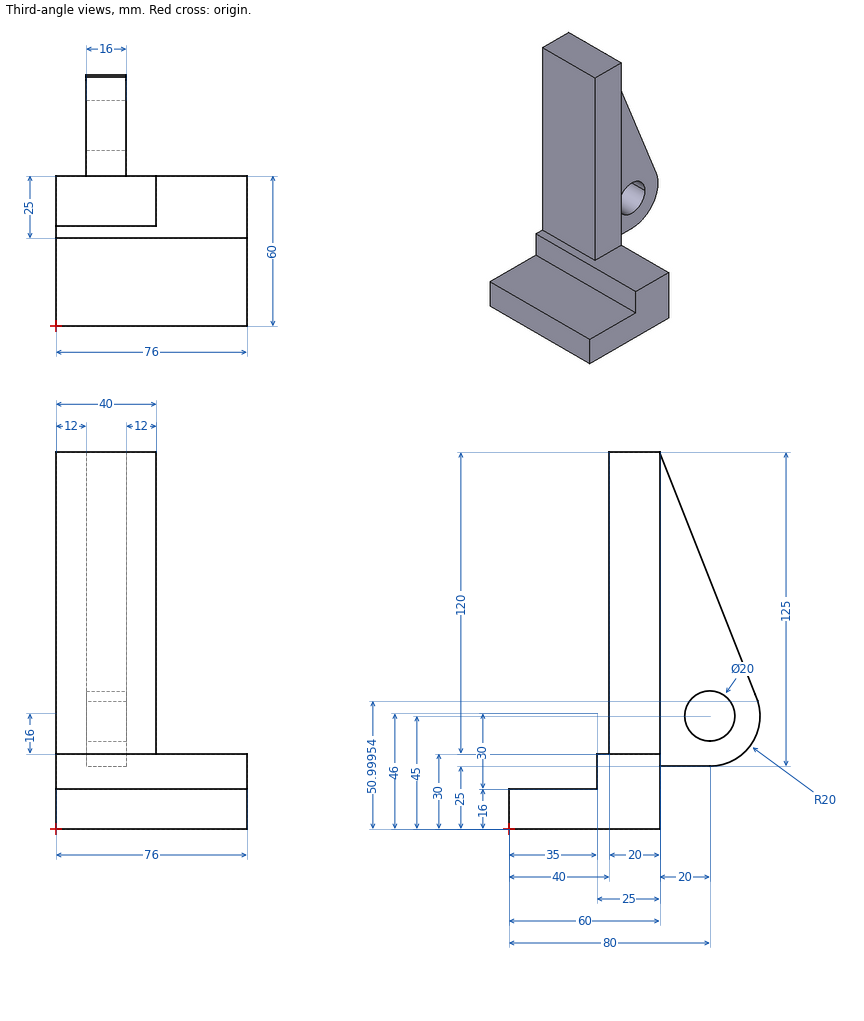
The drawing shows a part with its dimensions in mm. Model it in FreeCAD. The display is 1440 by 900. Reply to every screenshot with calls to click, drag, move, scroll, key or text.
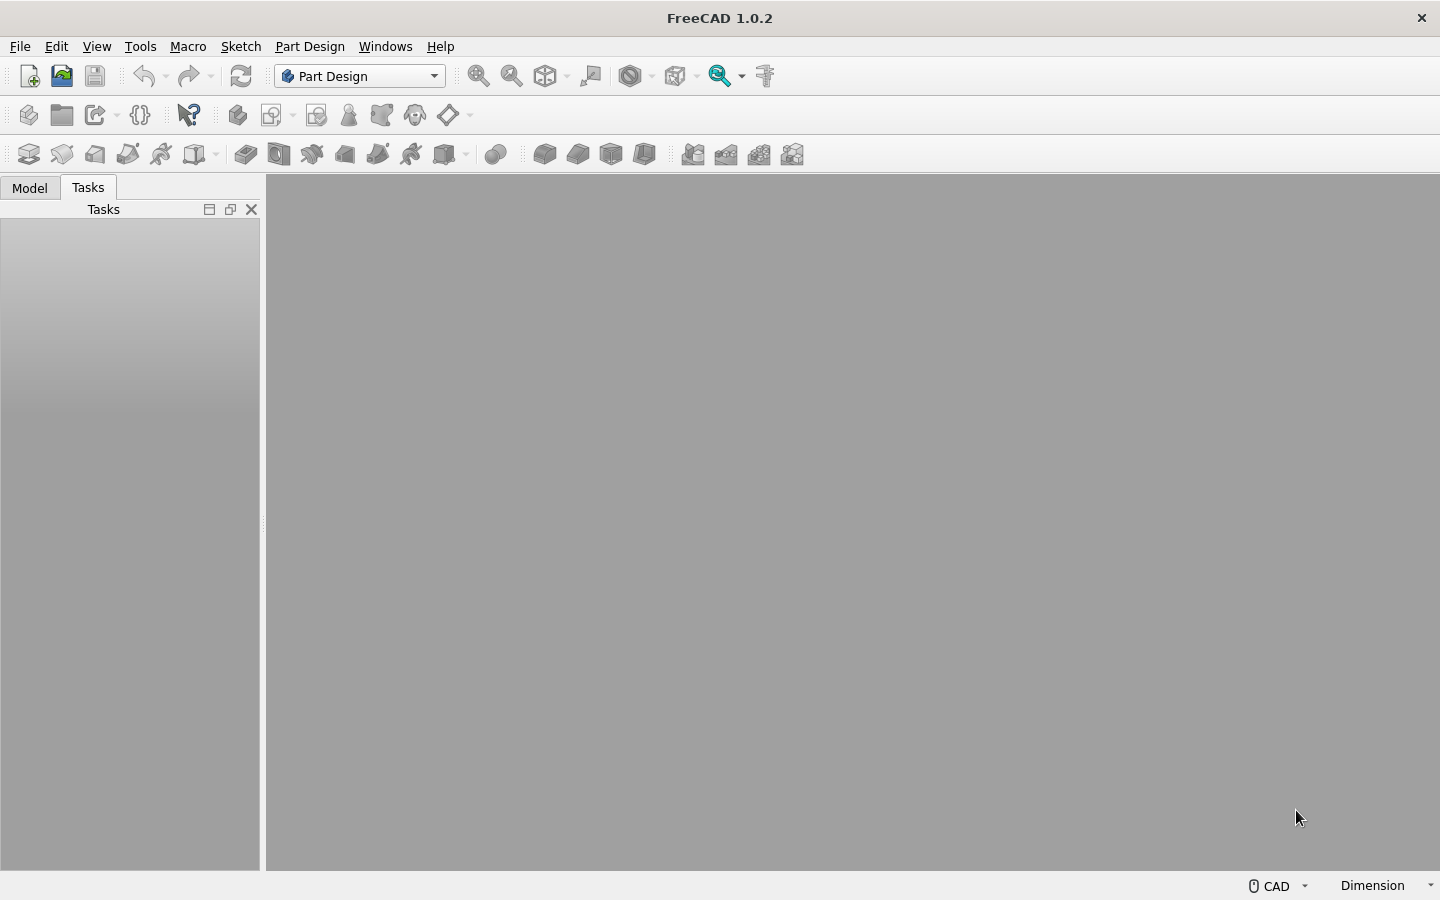
key(ctrl+n)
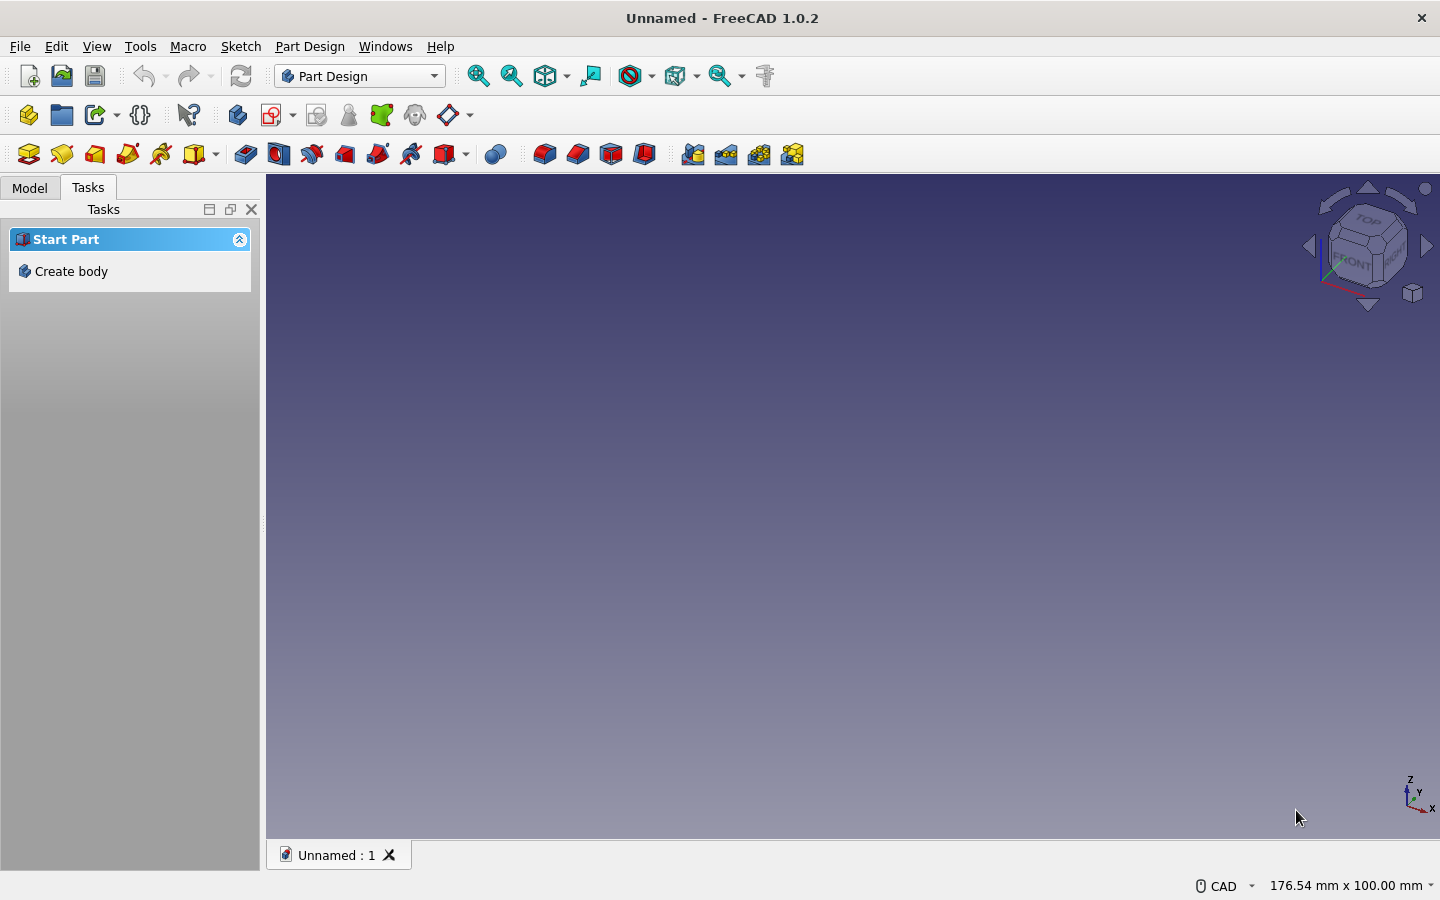
click(270, 116)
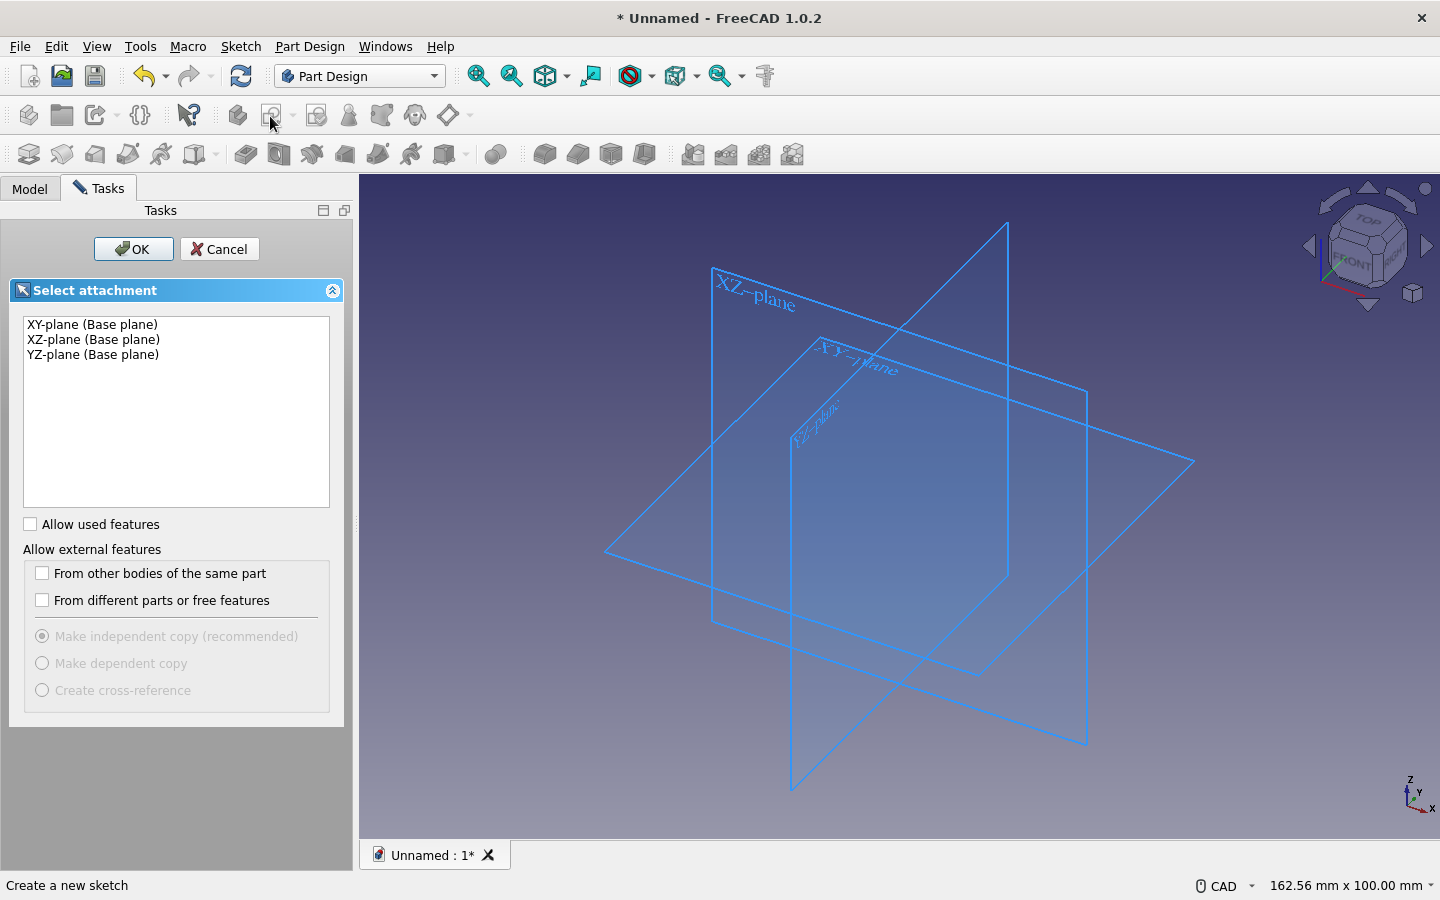
click(84, 324)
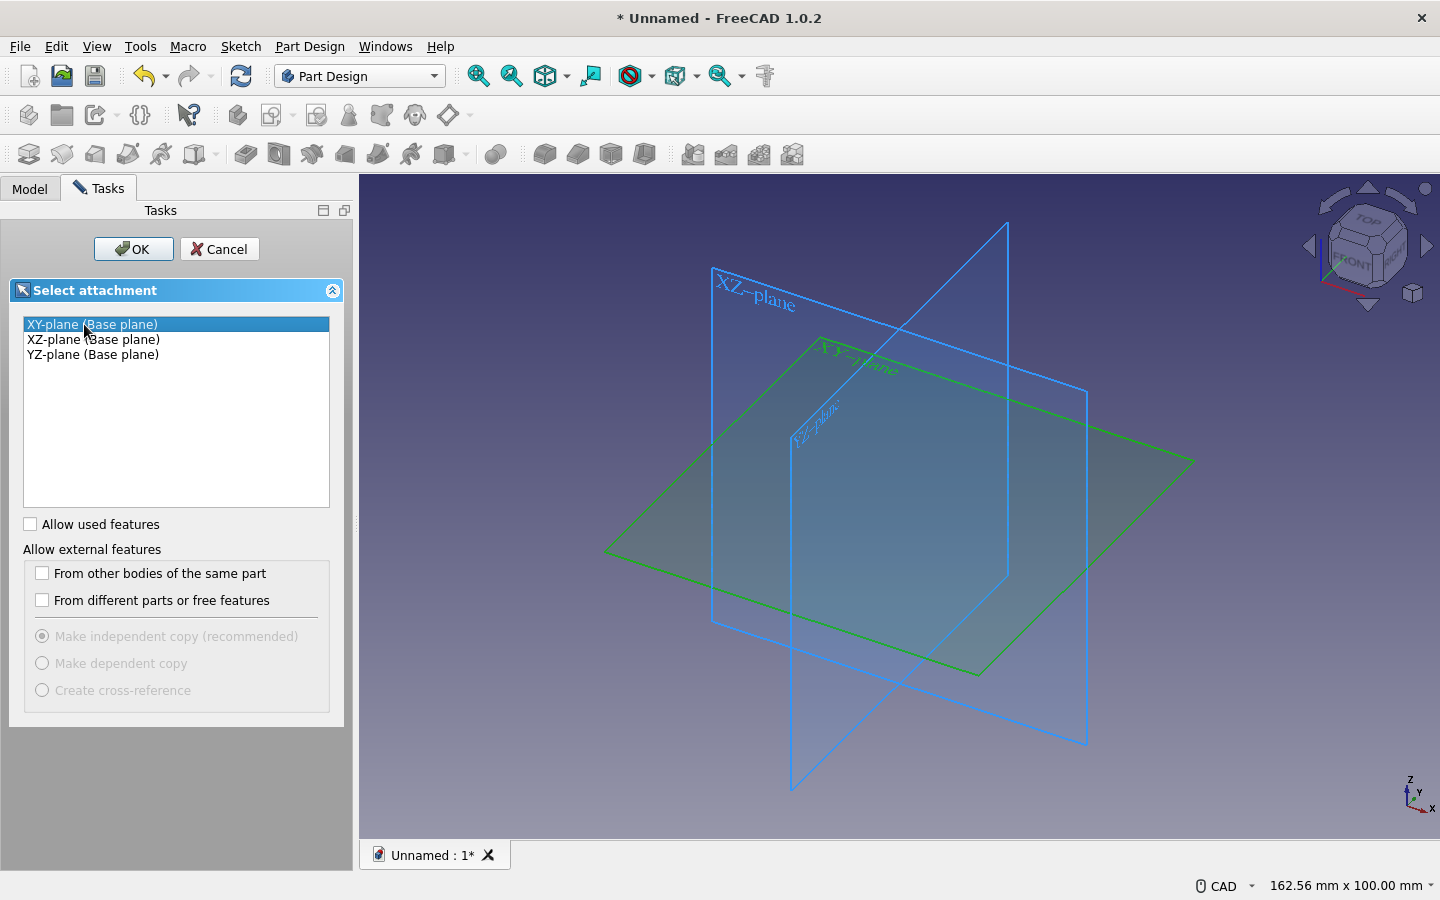
click(134, 249)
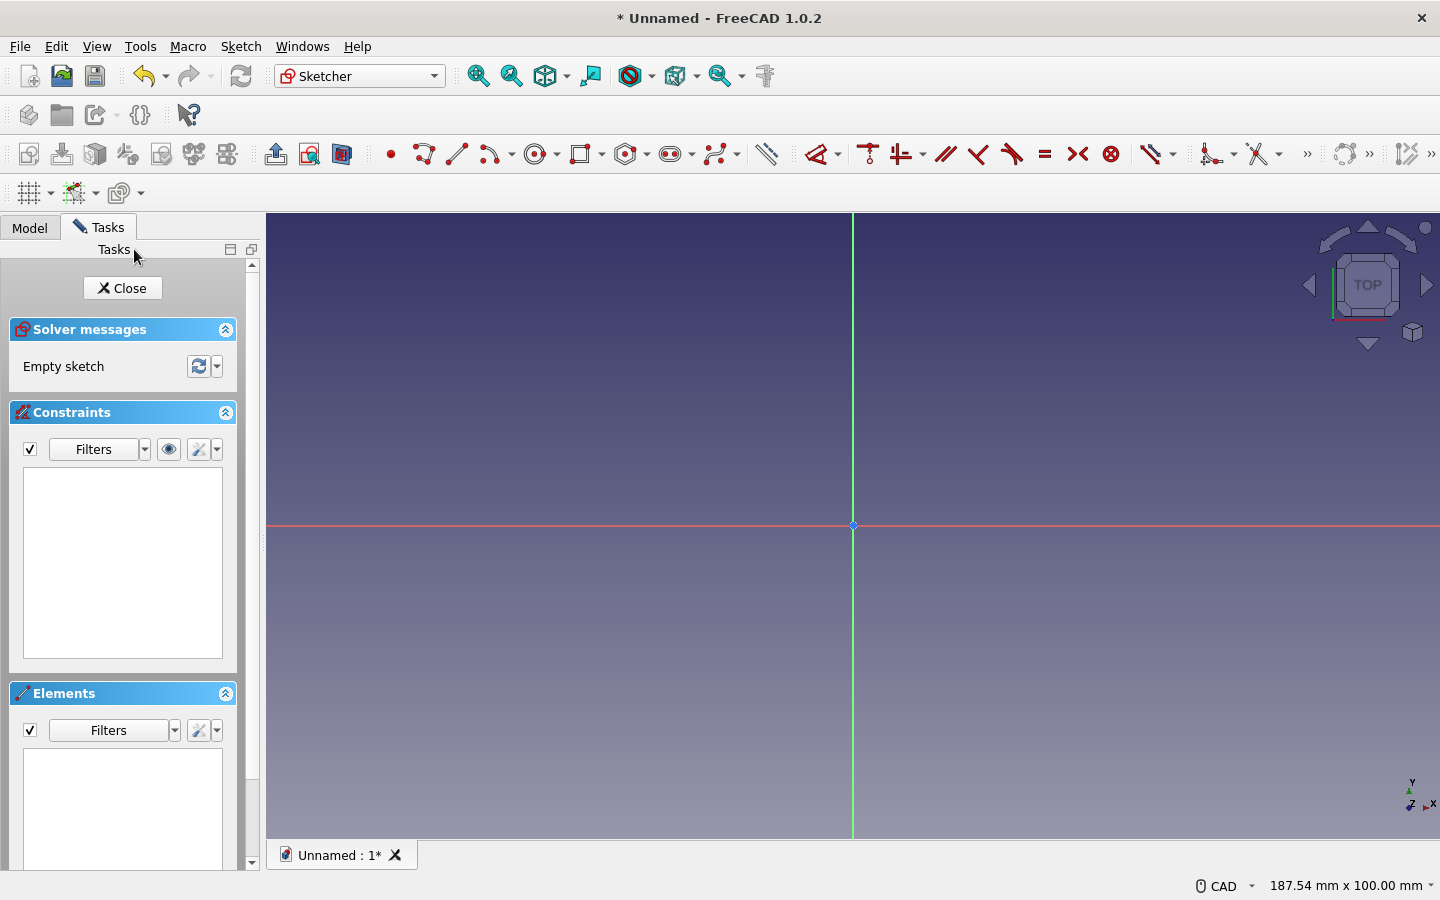
scroll(294, 811, down, 1)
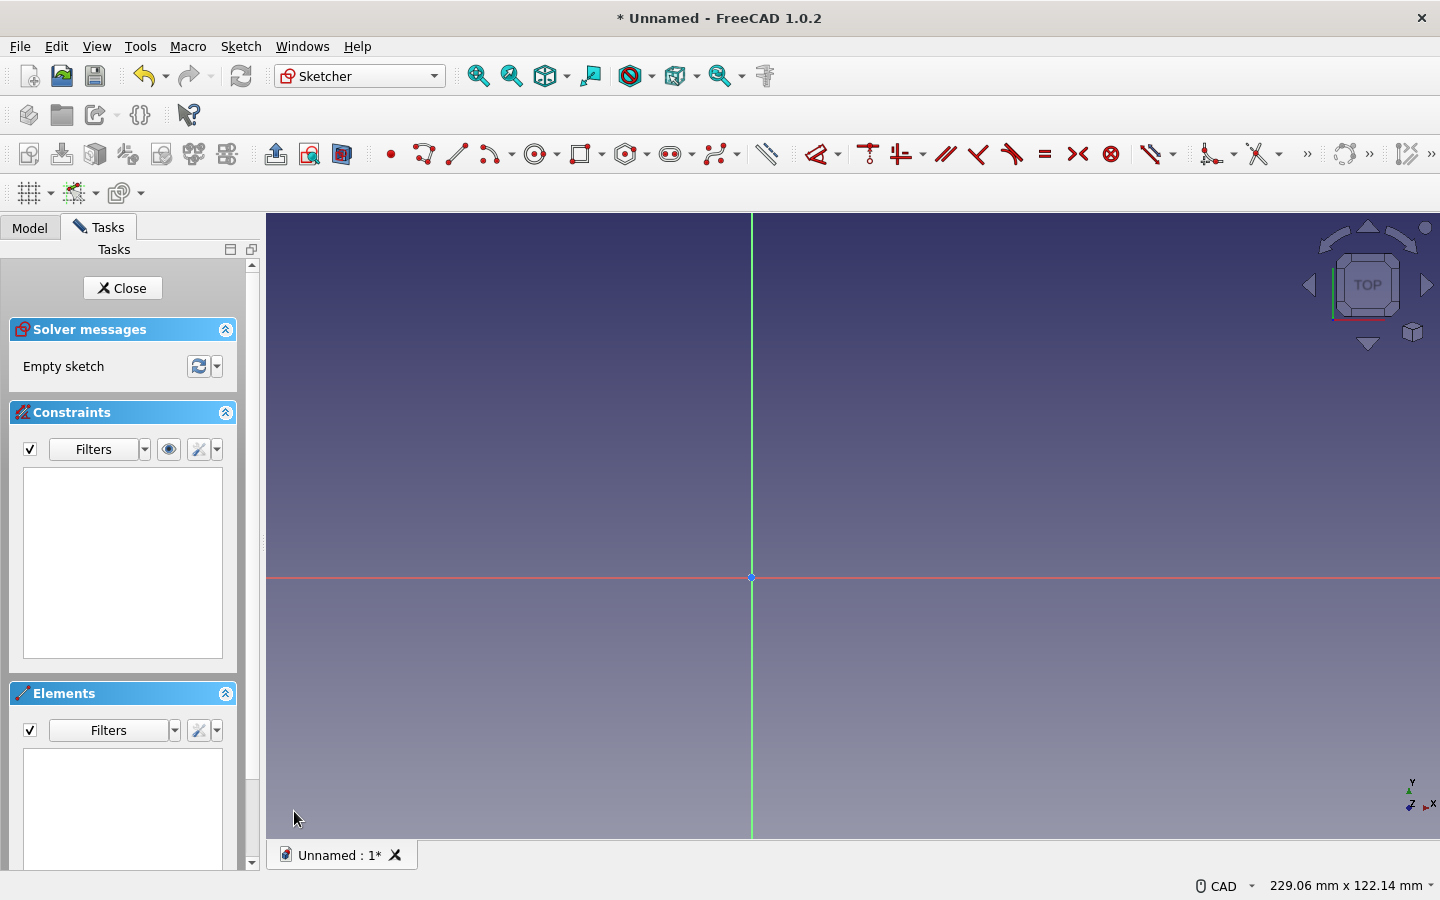
key(g)
key(r)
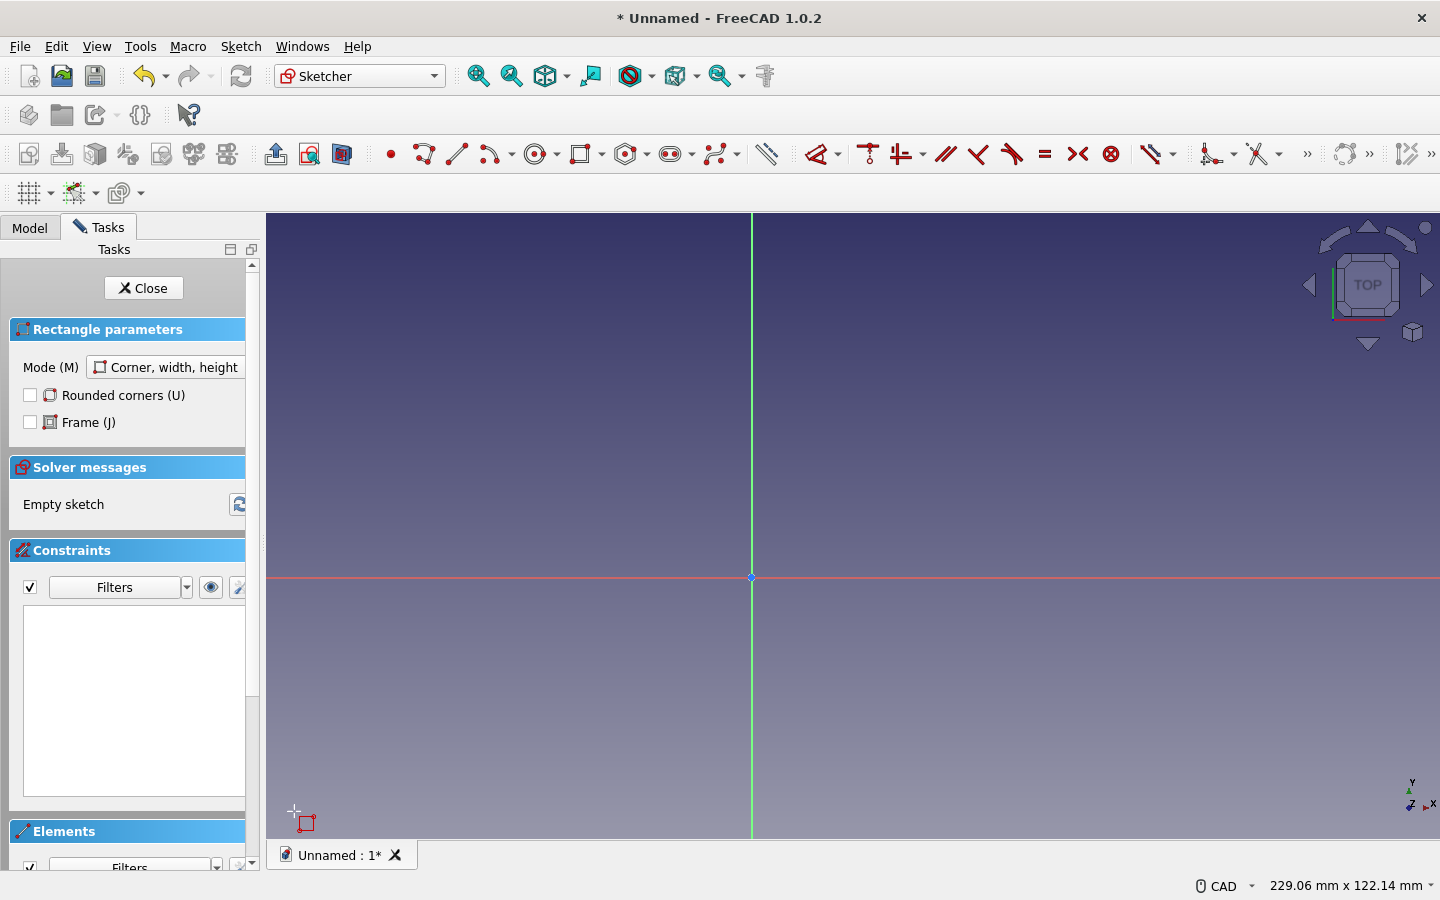
click(752, 578)
click(1141, 270)
key(Escape)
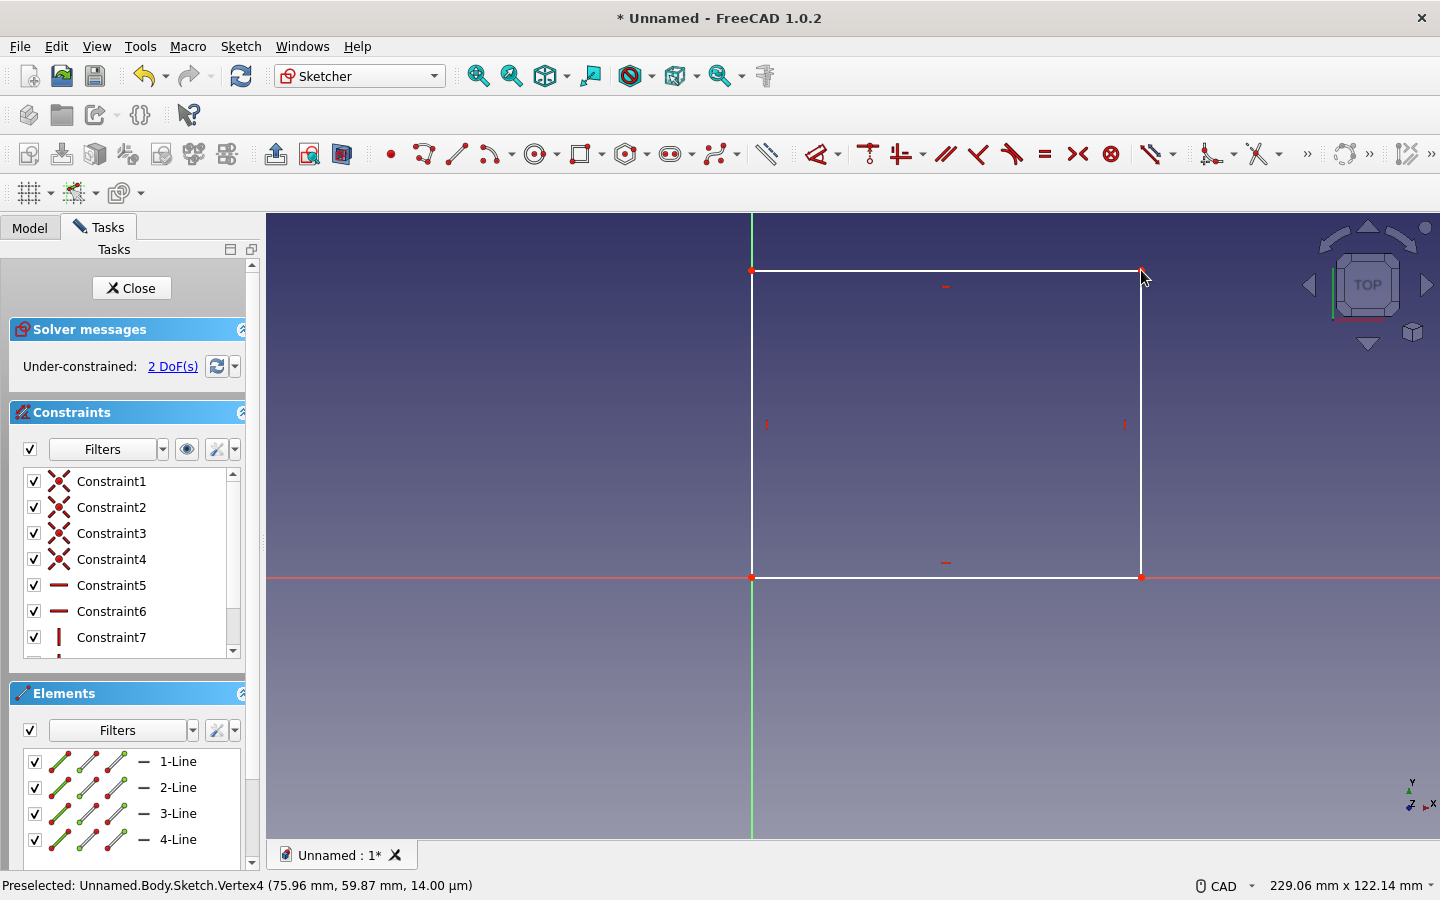
key(d)